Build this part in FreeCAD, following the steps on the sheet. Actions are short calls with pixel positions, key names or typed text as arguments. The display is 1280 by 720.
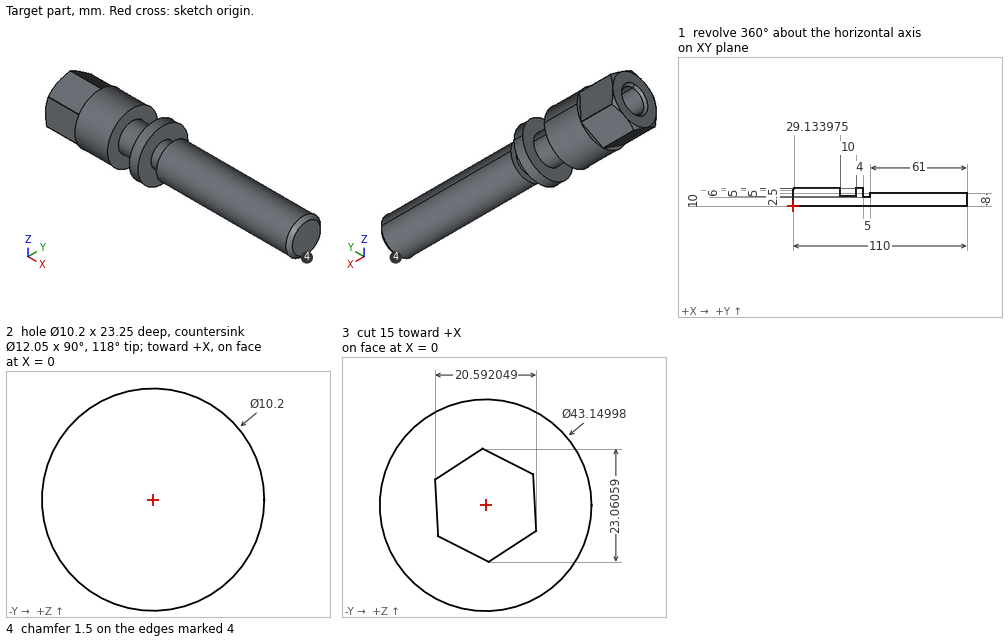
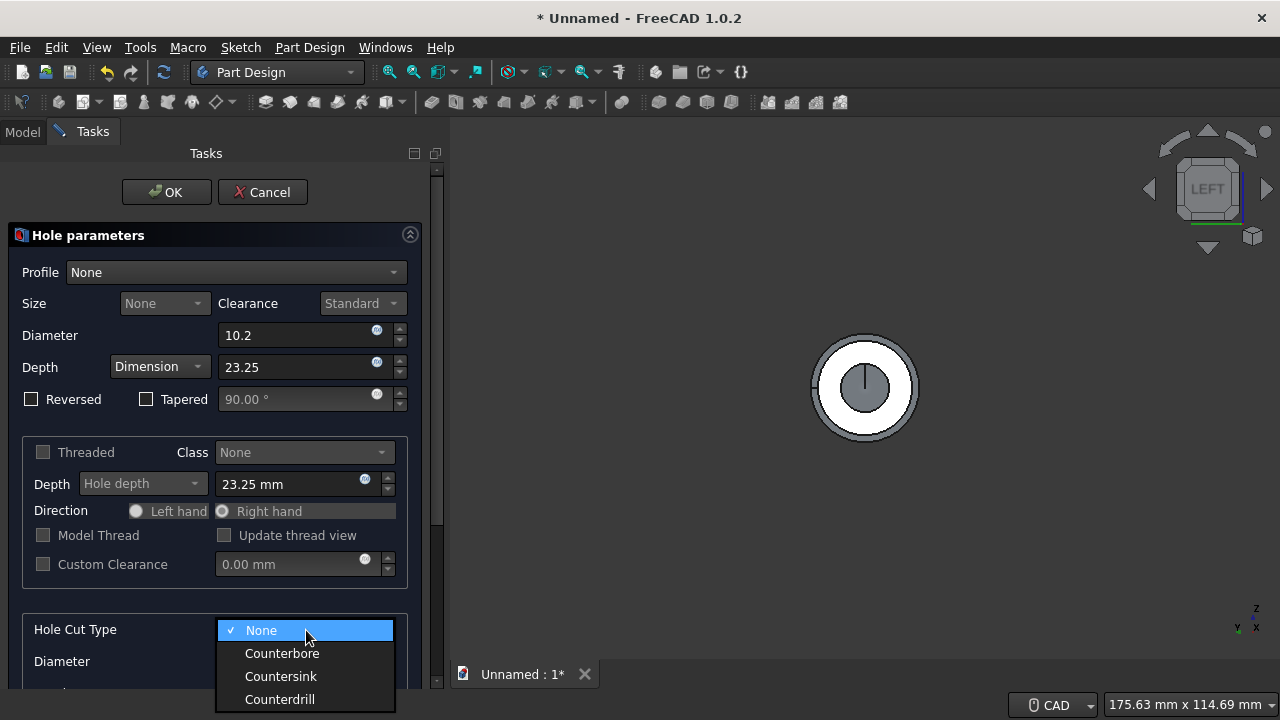
click(304, 676)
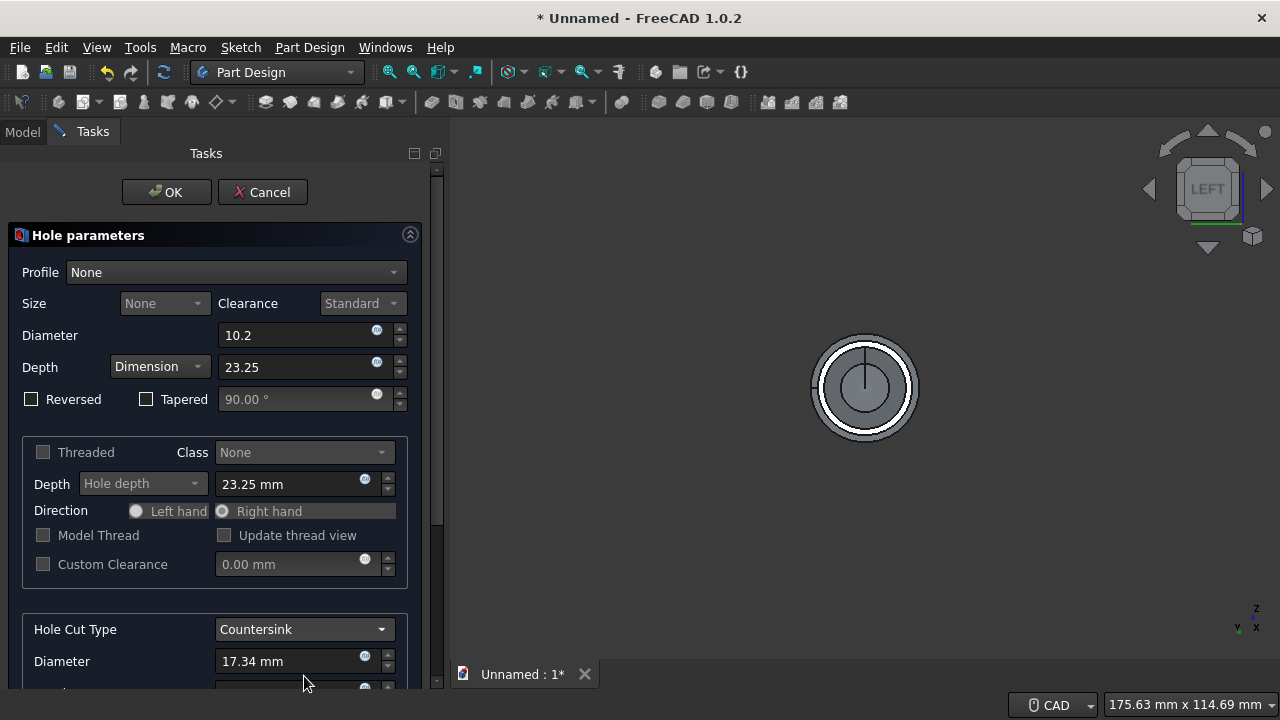
triple_click(298, 661)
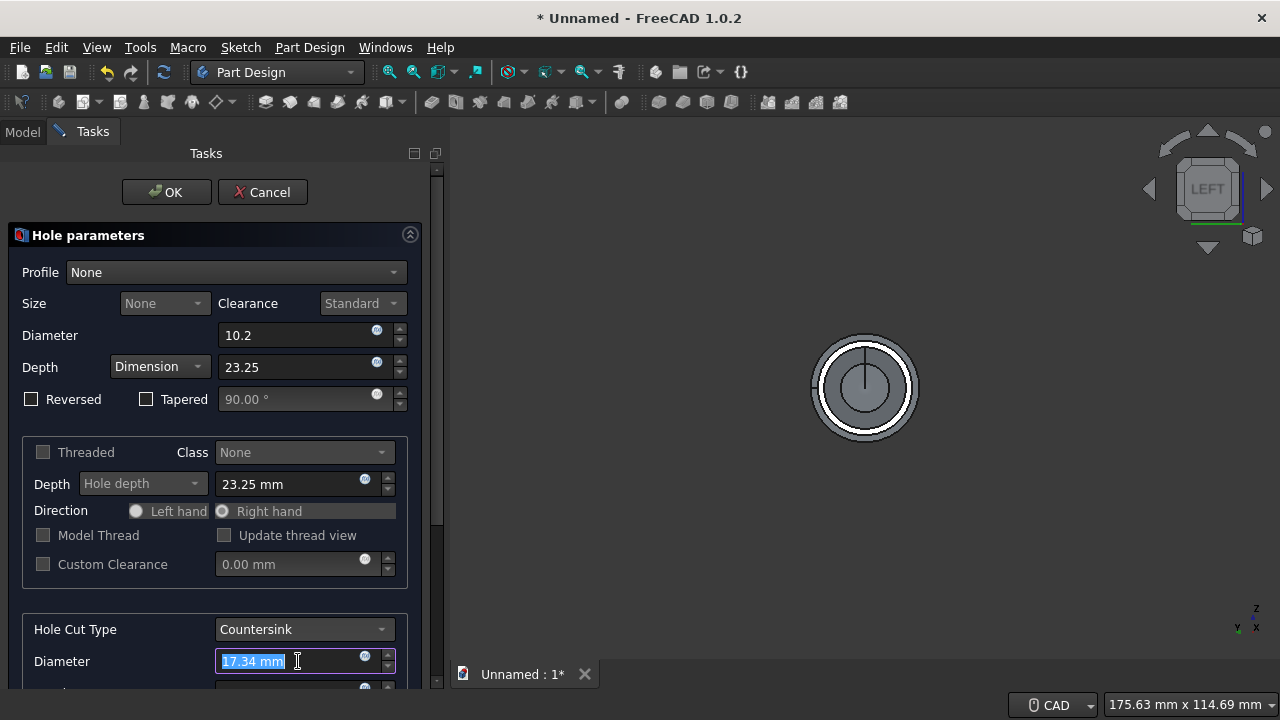
text(12.05)
key(Tab)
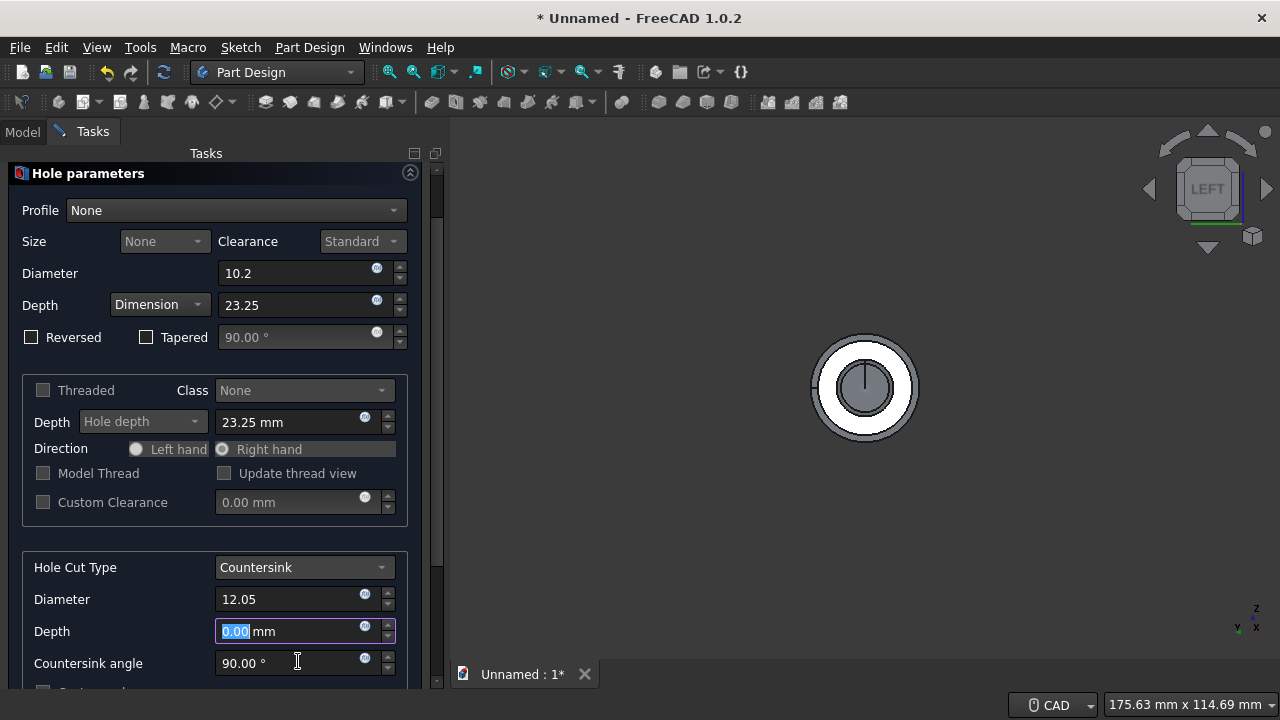
scroll(437, 426, up, 2)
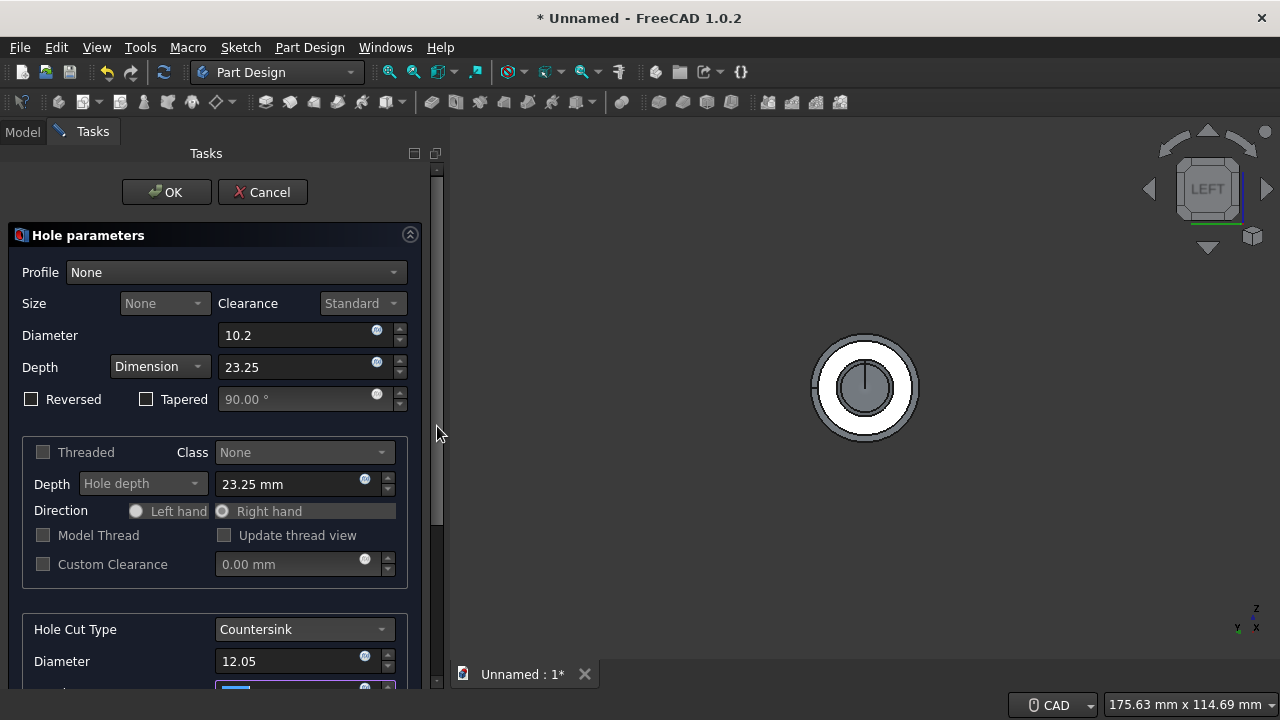
click(167, 192)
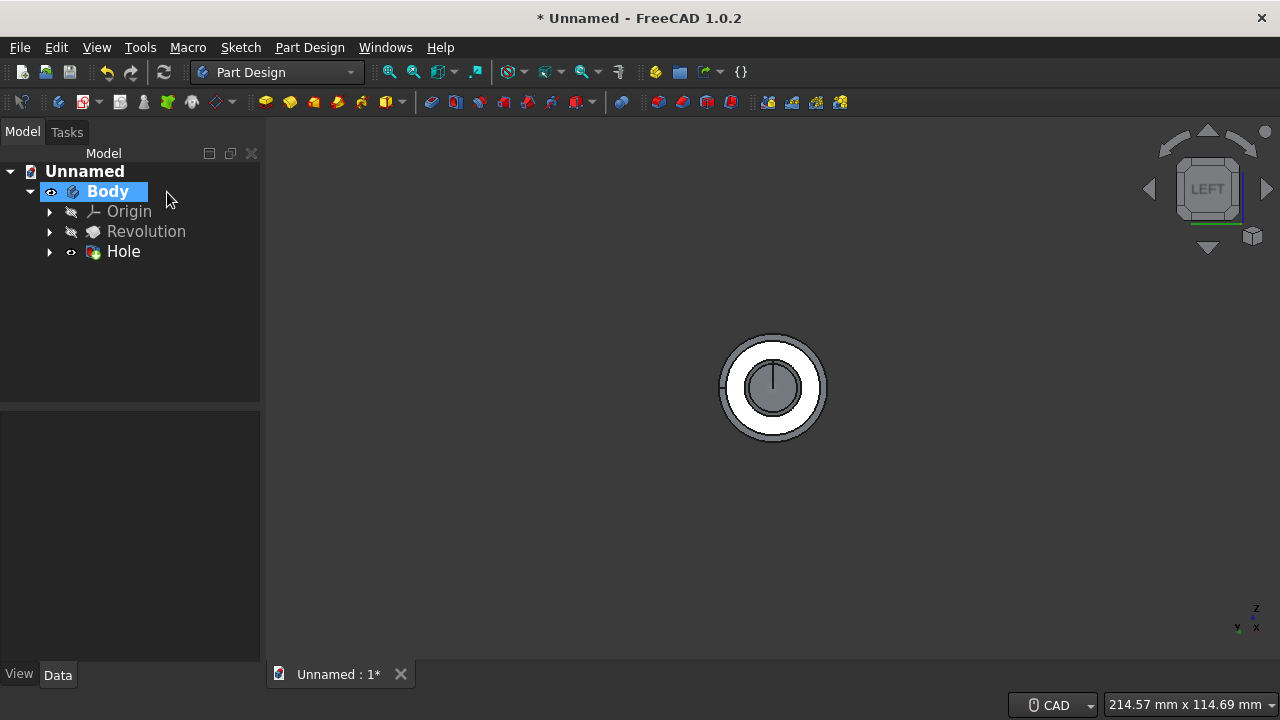
key(v)
key(f)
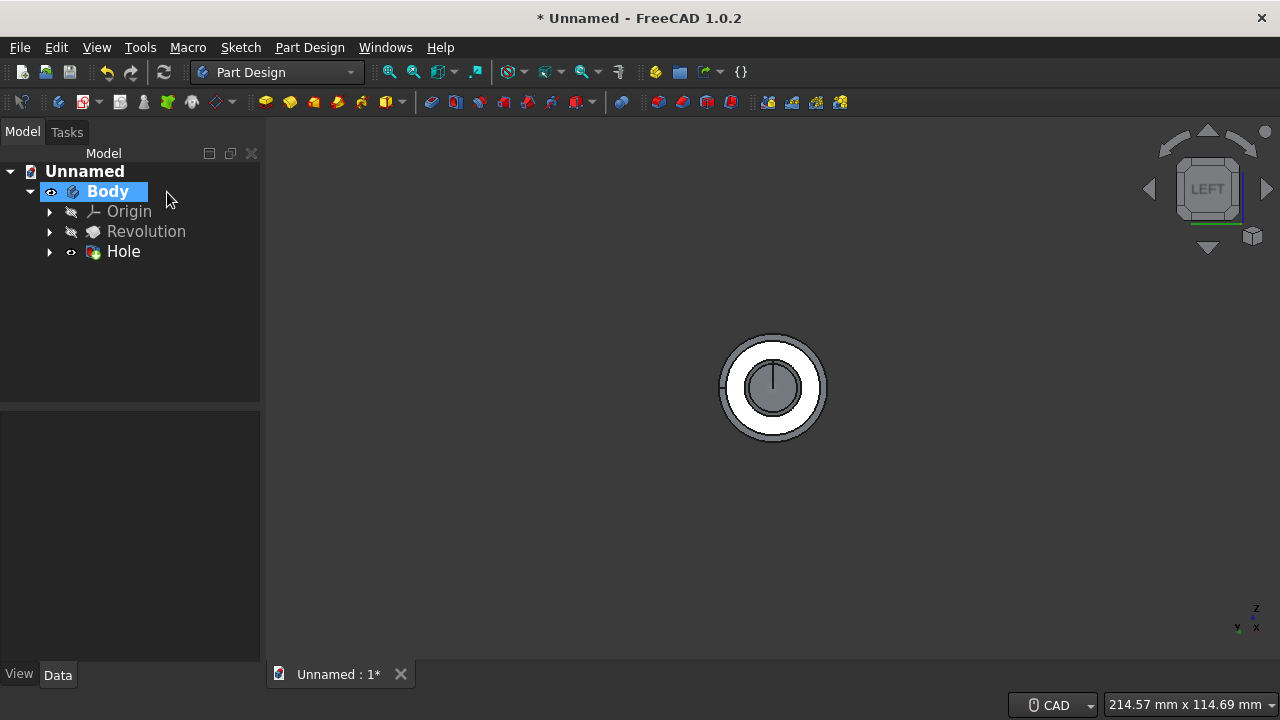
click(746, 360)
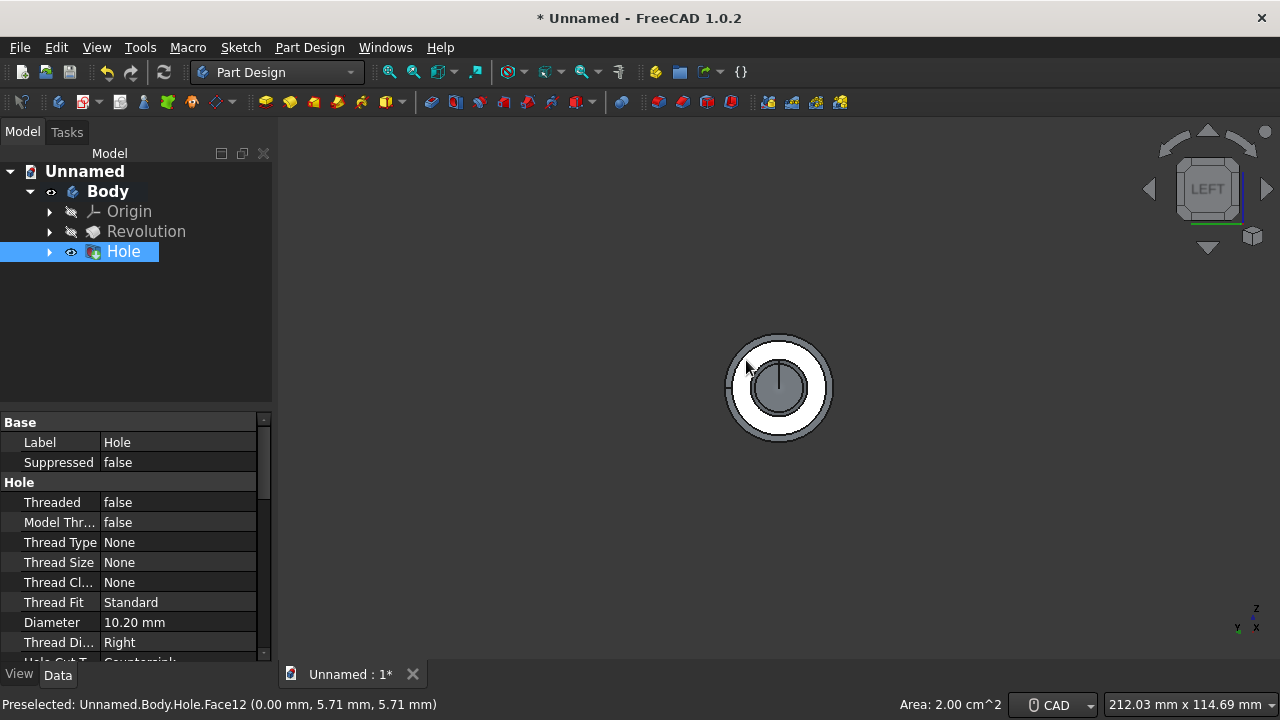
click(84, 102)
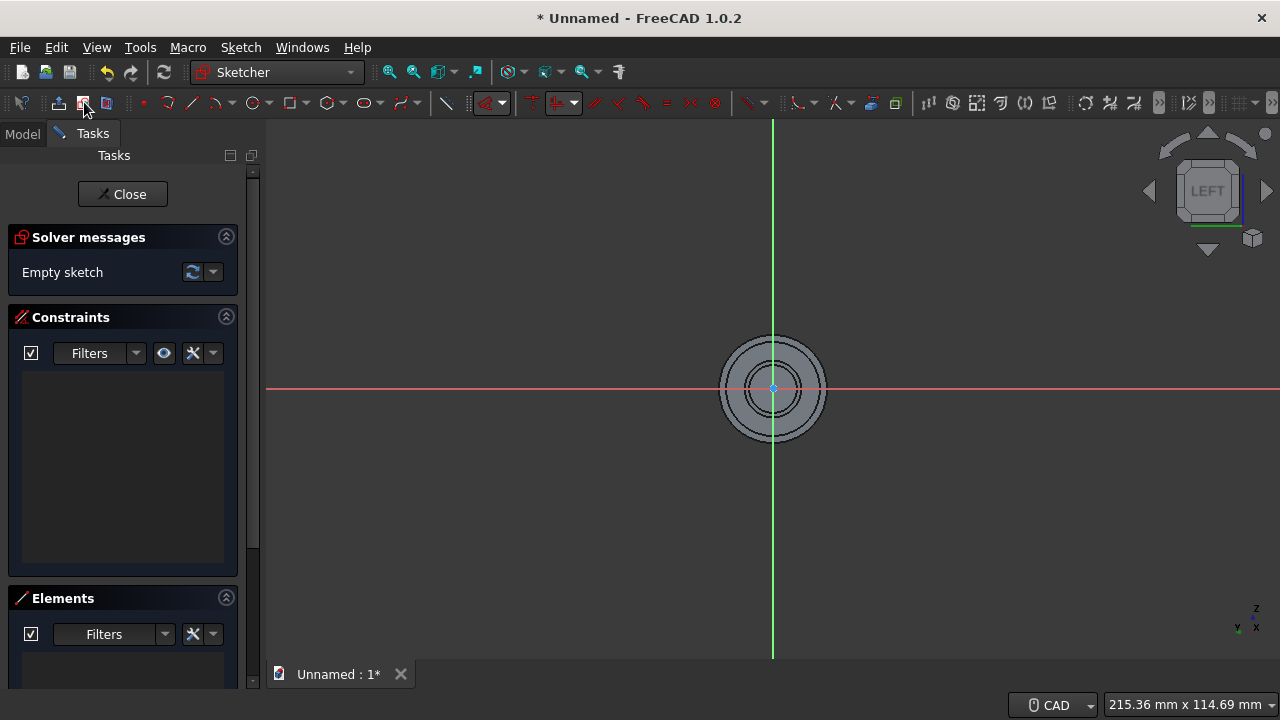
scroll(856, 389, up, 3)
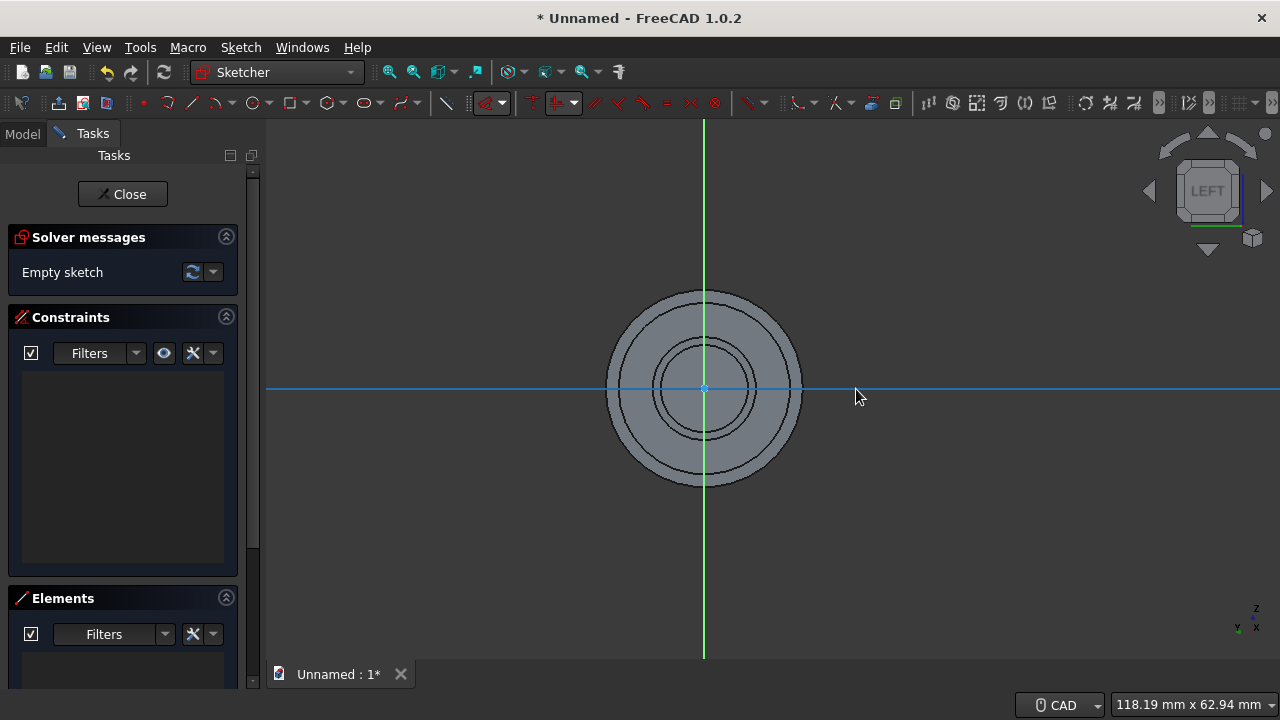
key(g)
key(p)
key(6)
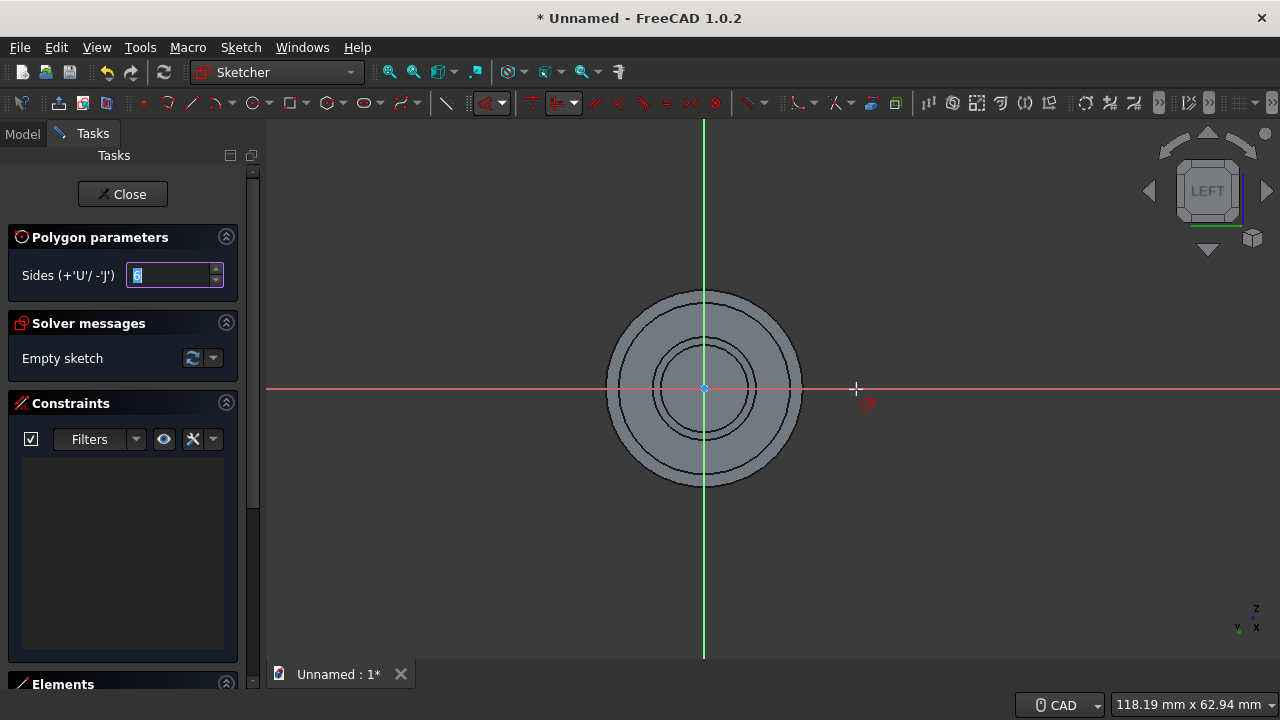
click(704, 389)